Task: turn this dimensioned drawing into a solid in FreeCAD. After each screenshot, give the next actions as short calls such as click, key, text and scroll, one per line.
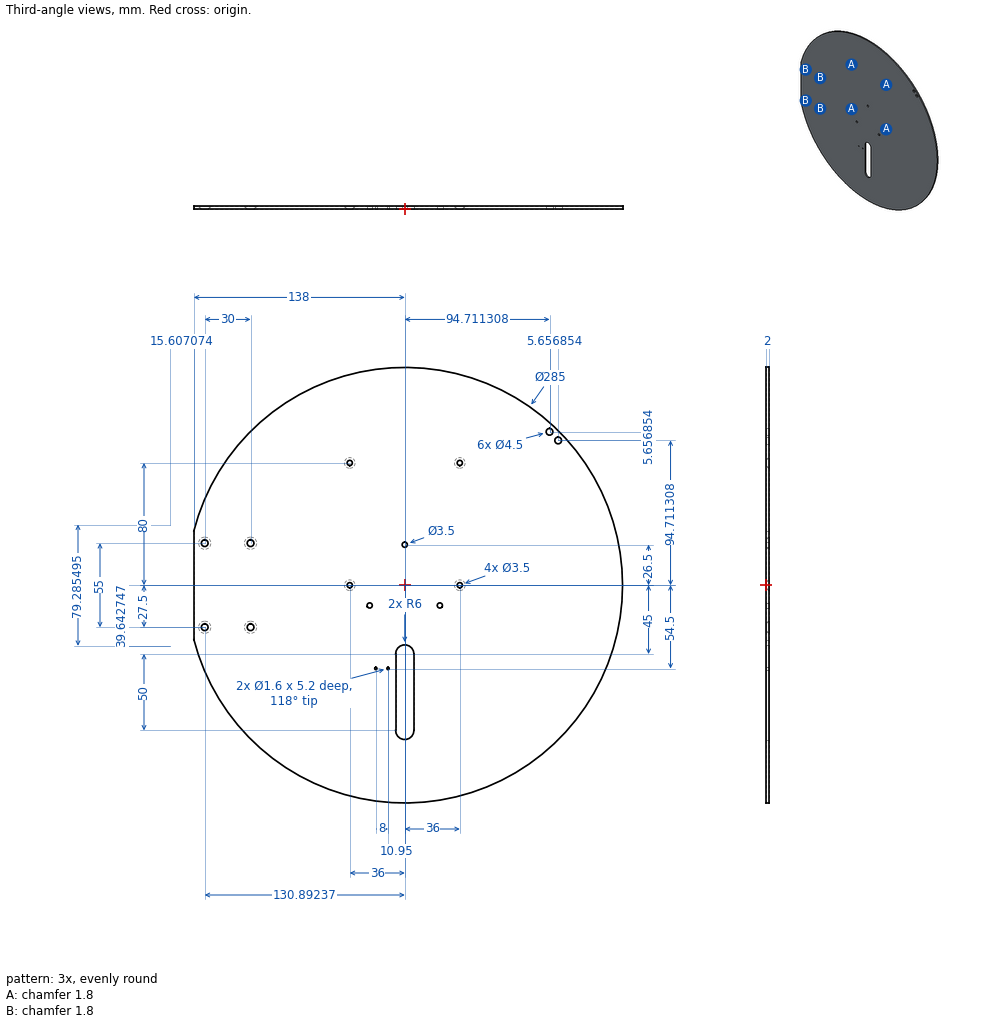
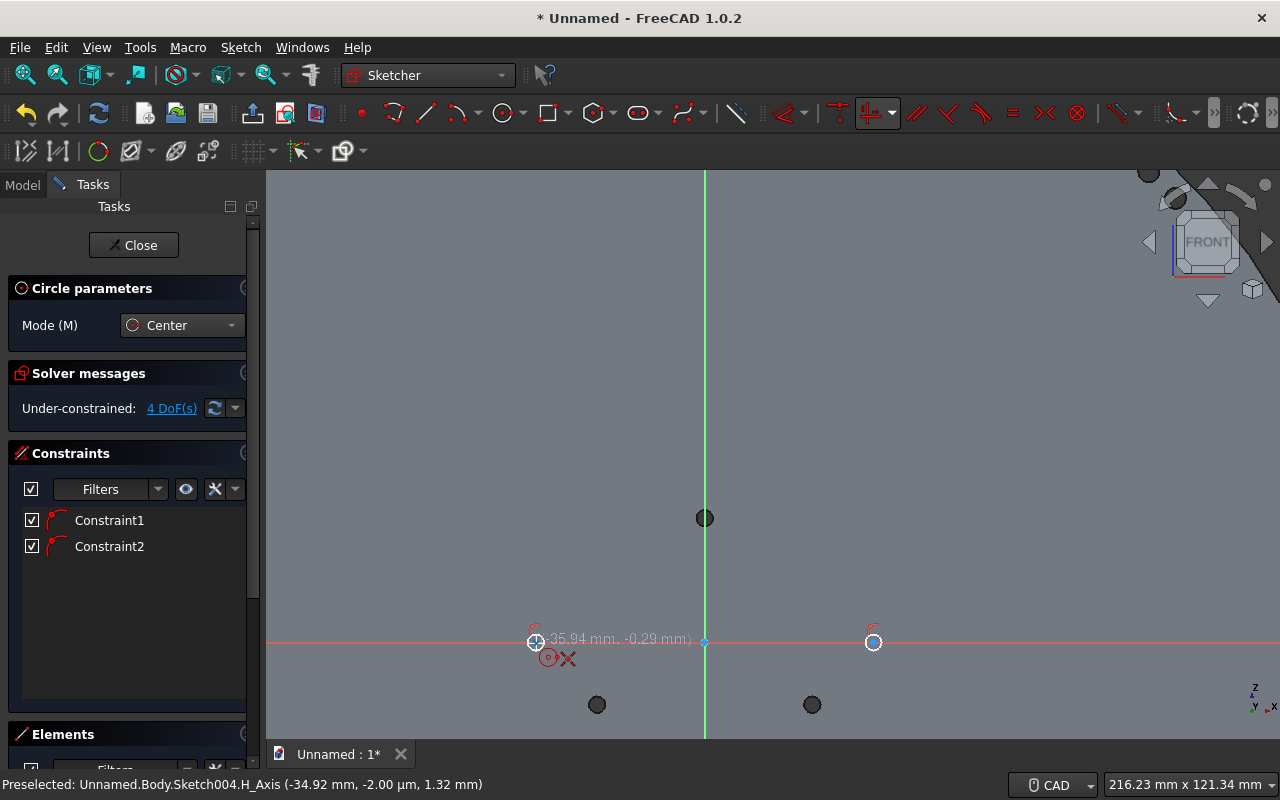
scroll(536, 267, up, 6)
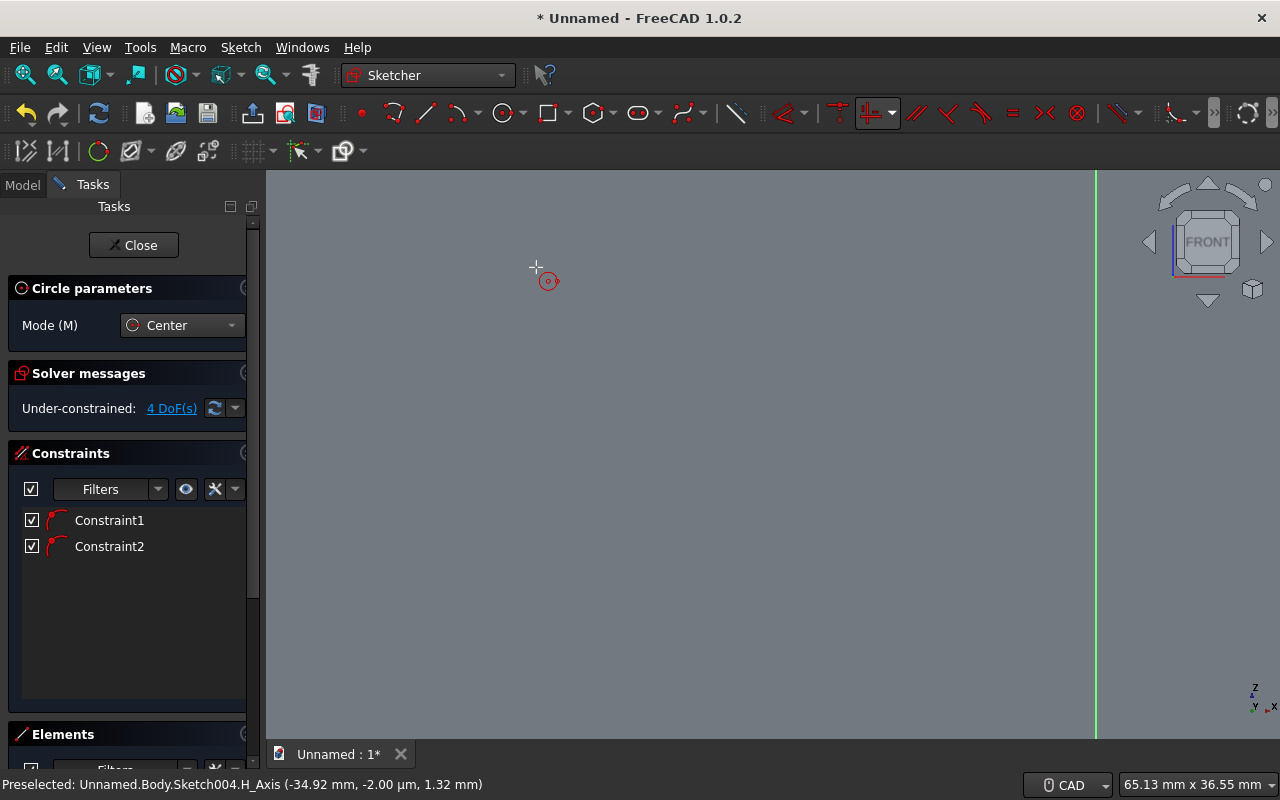
click(535, 268)
click(554, 249)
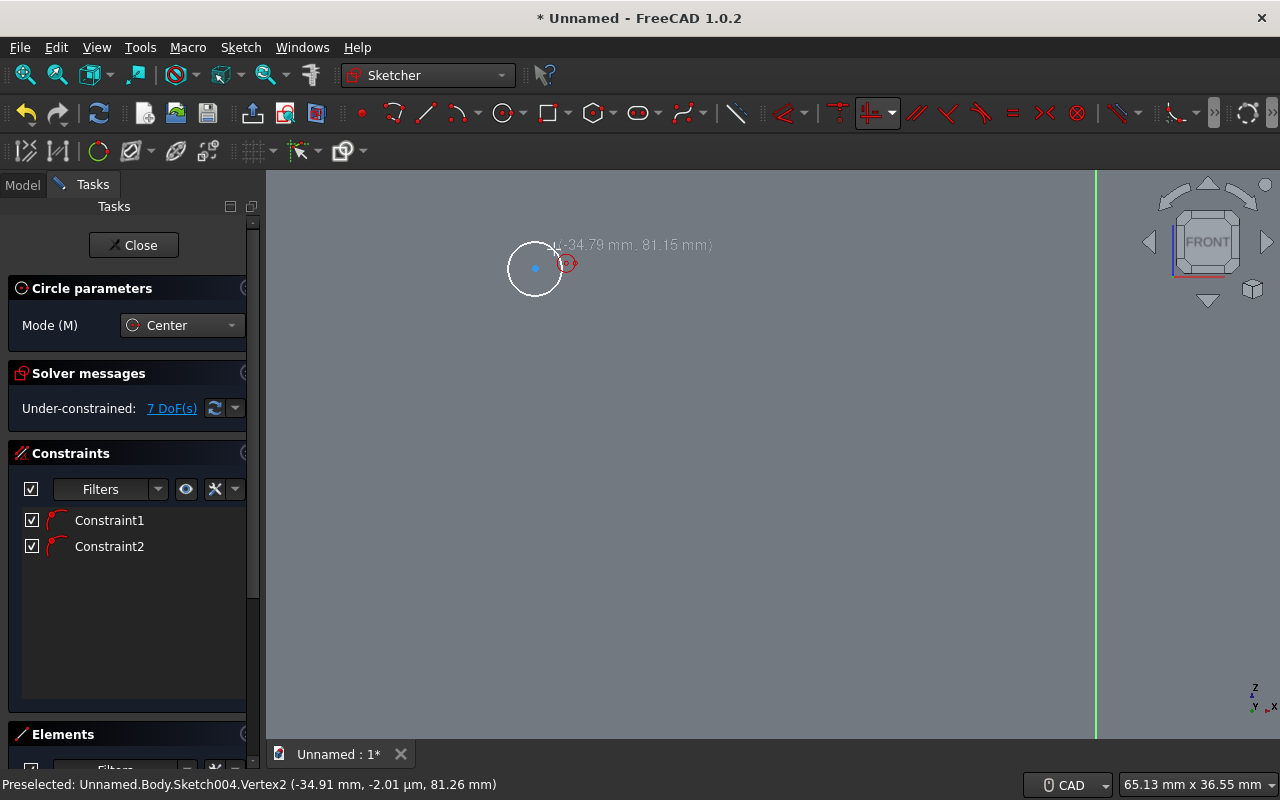
scroll(536, 267, down, 6)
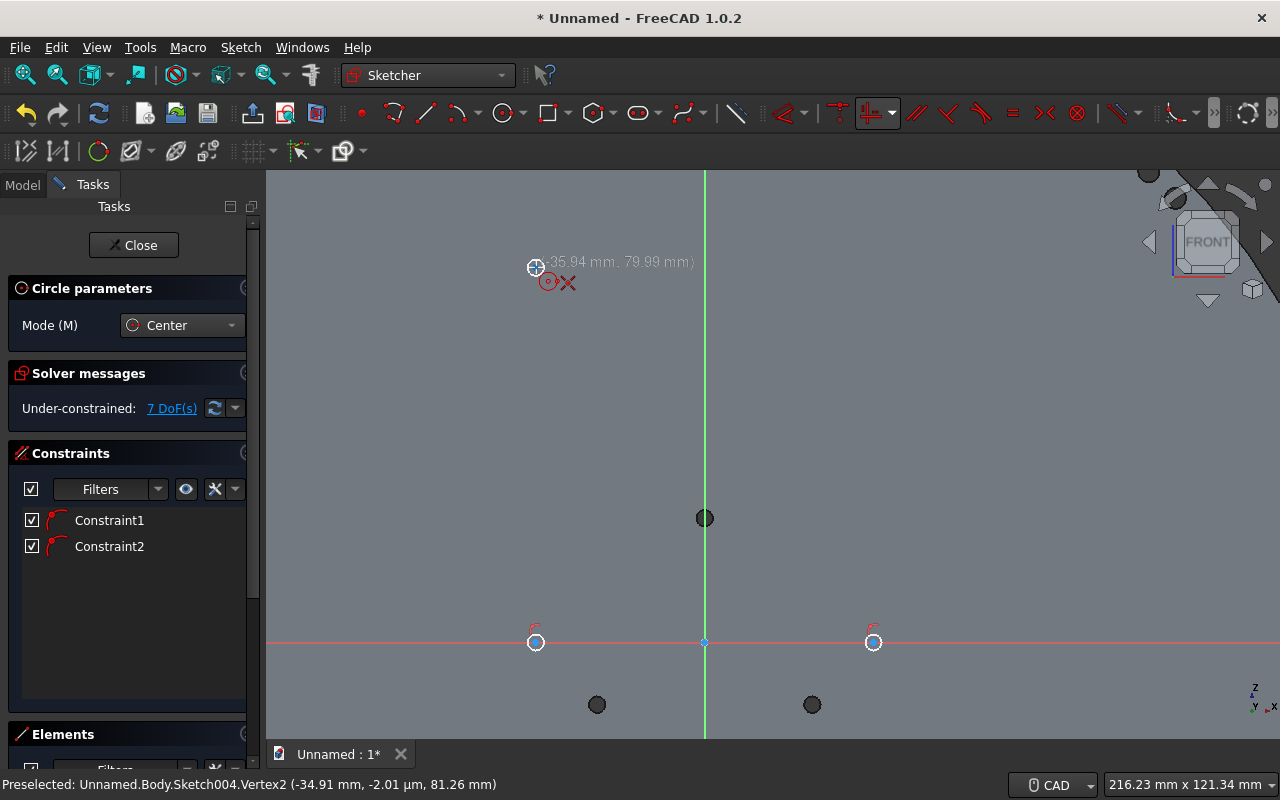
scroll(874, 267, up, 6)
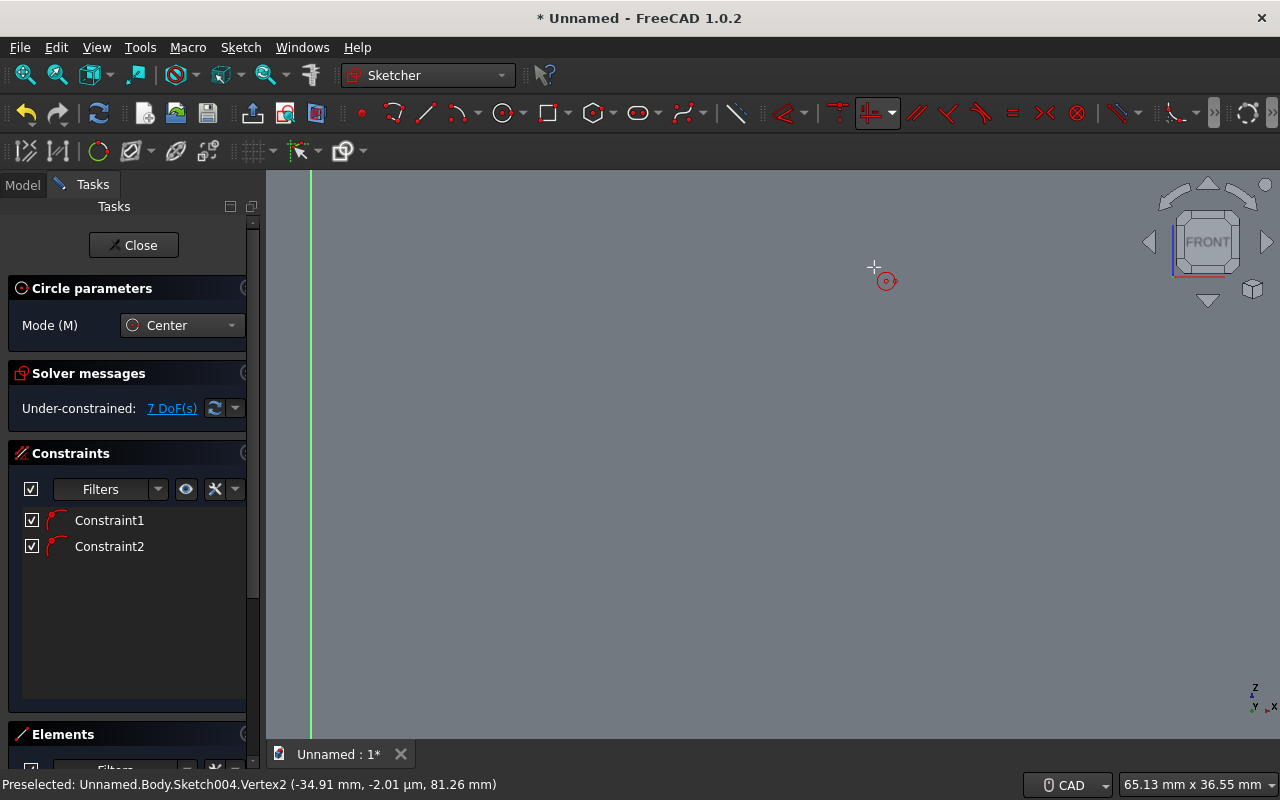
click(871, 268)
click(890, 249)
key(Escape)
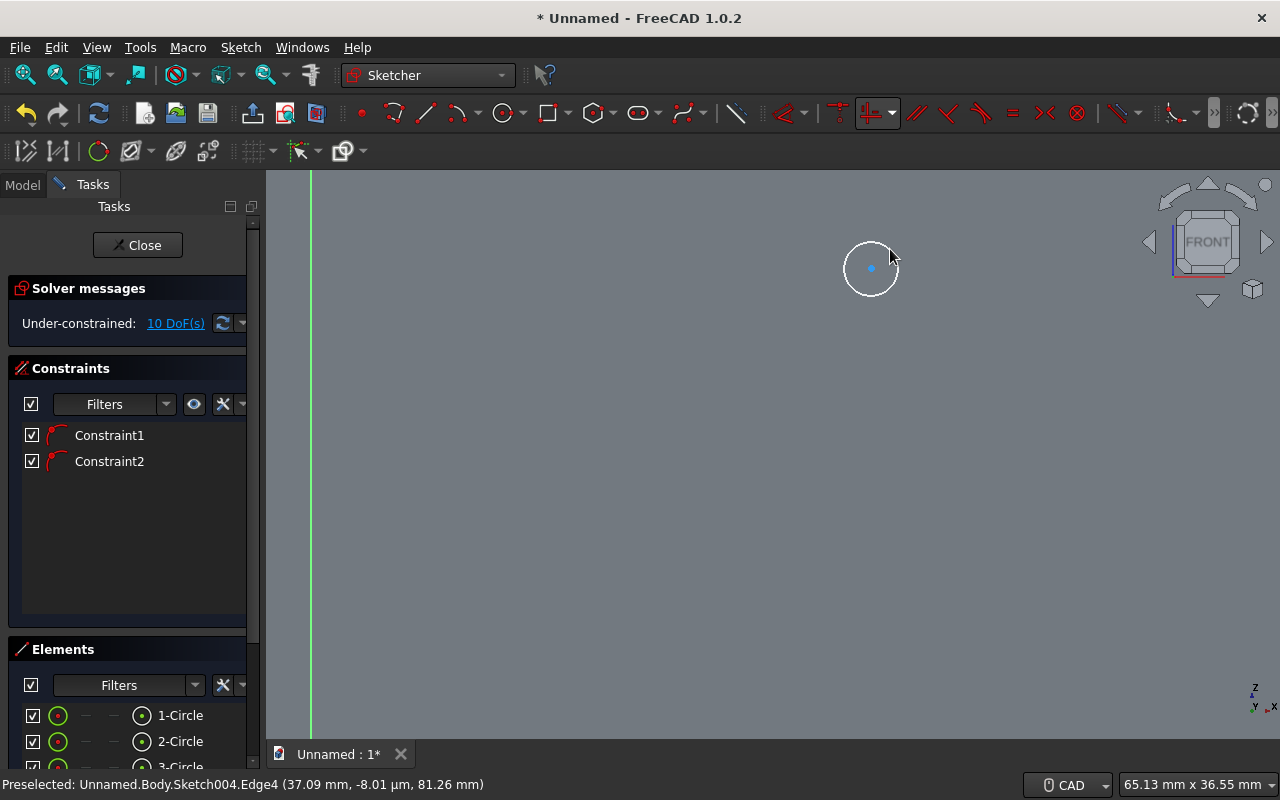
scroll(874, 267, down, 6)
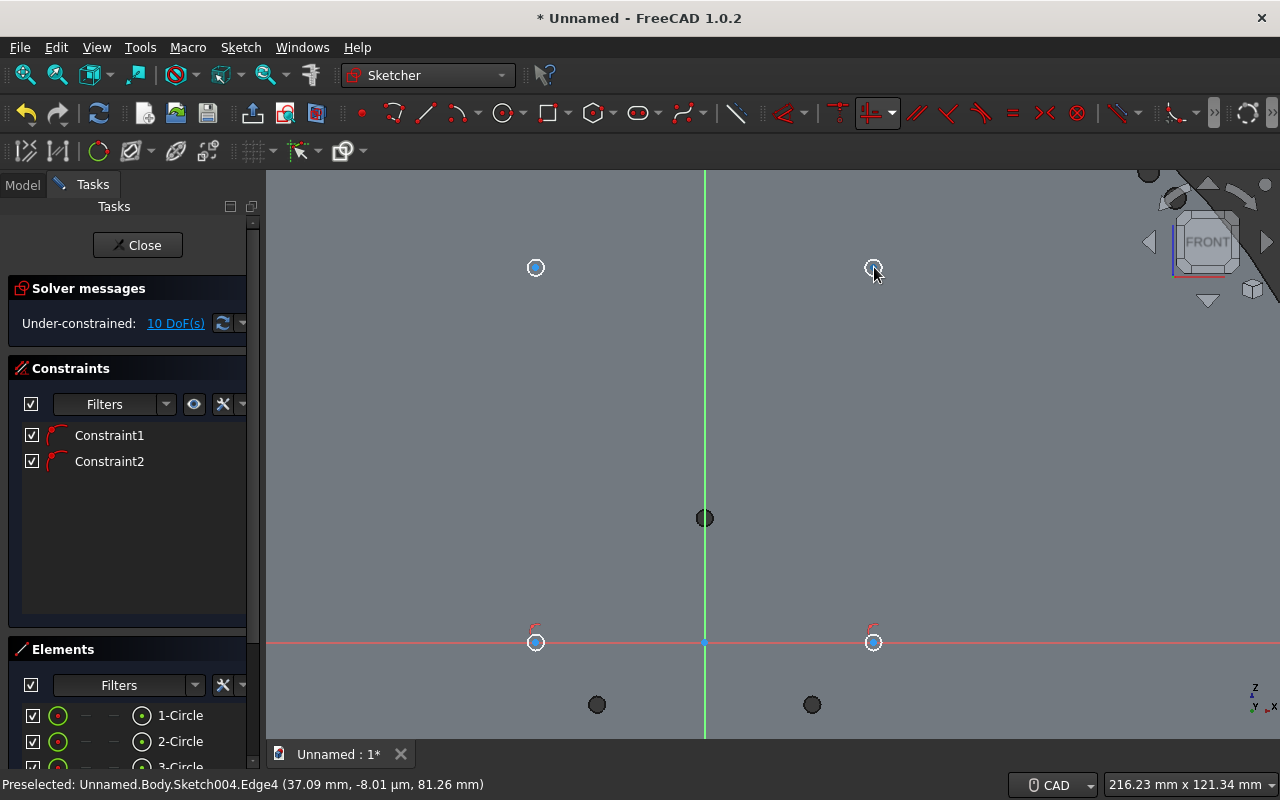
scroll(879, 637, up, 5)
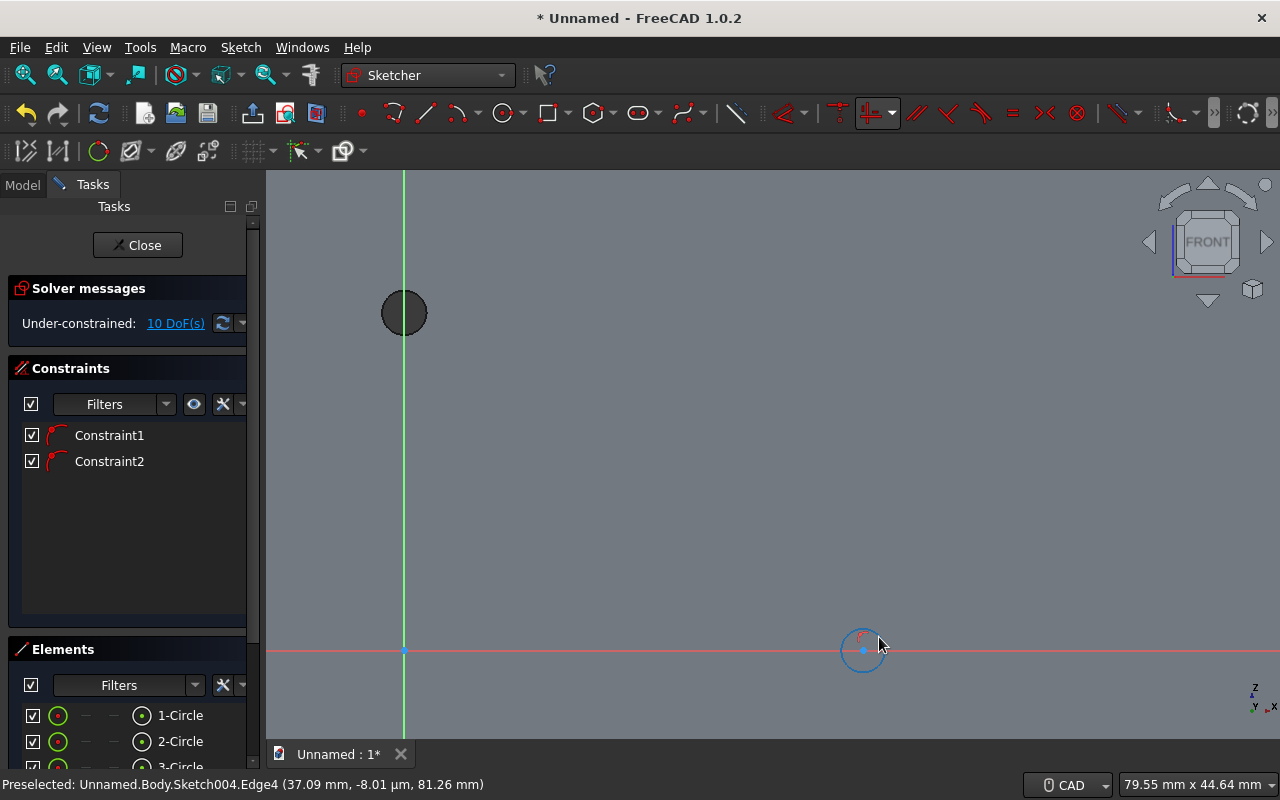
click(878, 635)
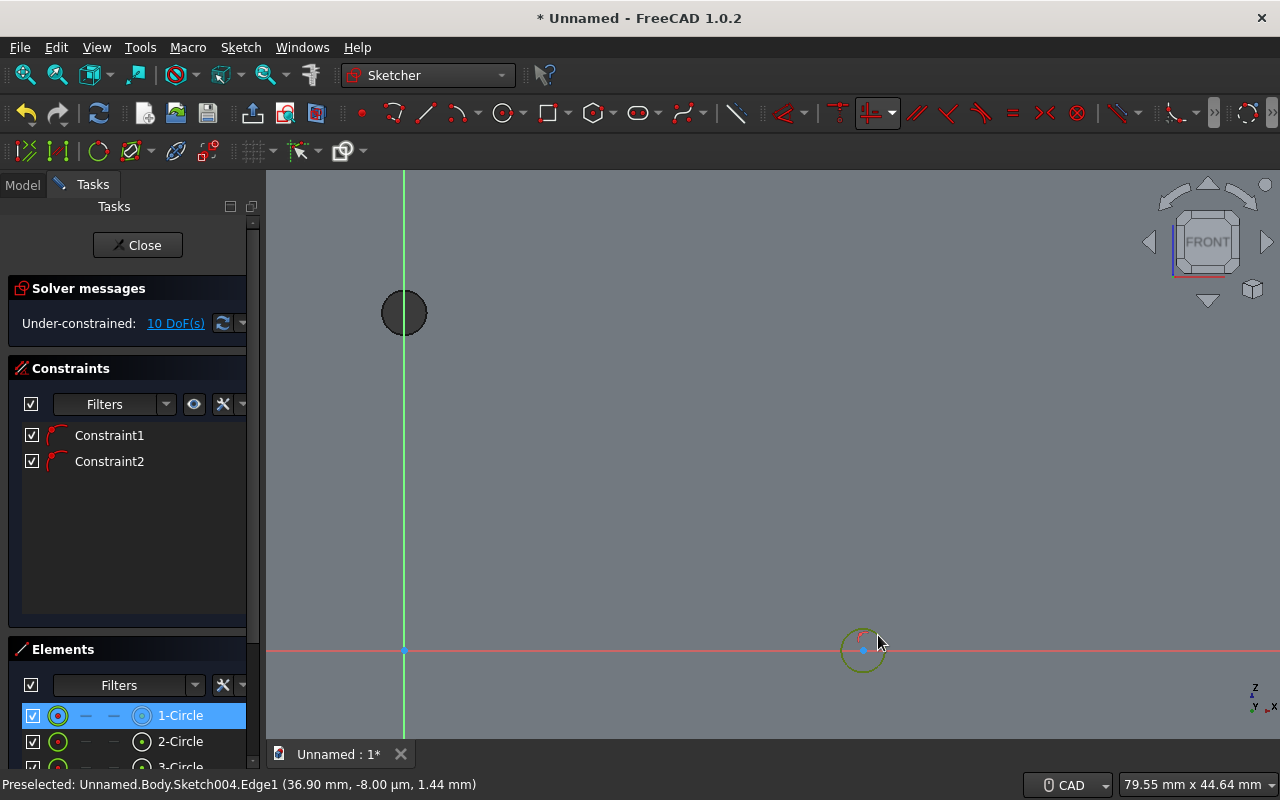
scroll(879, 637, down, 5)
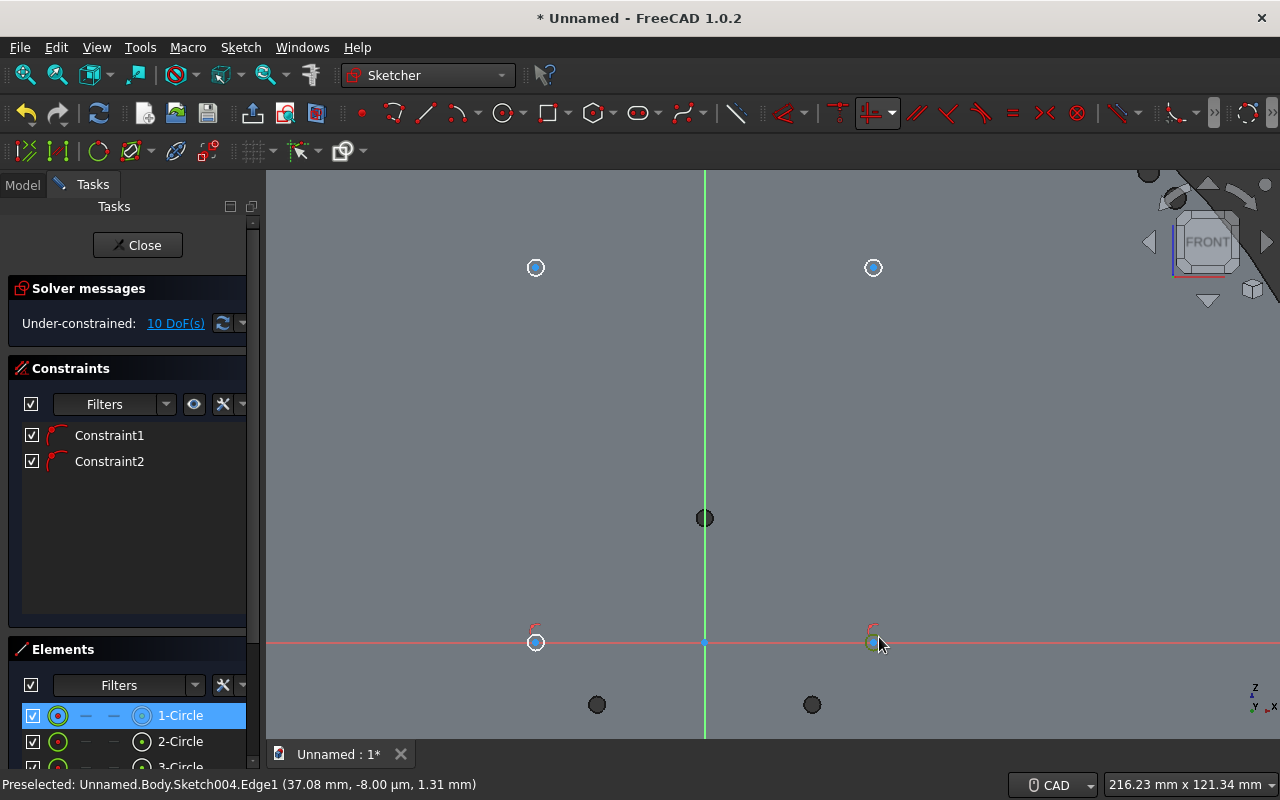
scroll(542, 637, up, 5)